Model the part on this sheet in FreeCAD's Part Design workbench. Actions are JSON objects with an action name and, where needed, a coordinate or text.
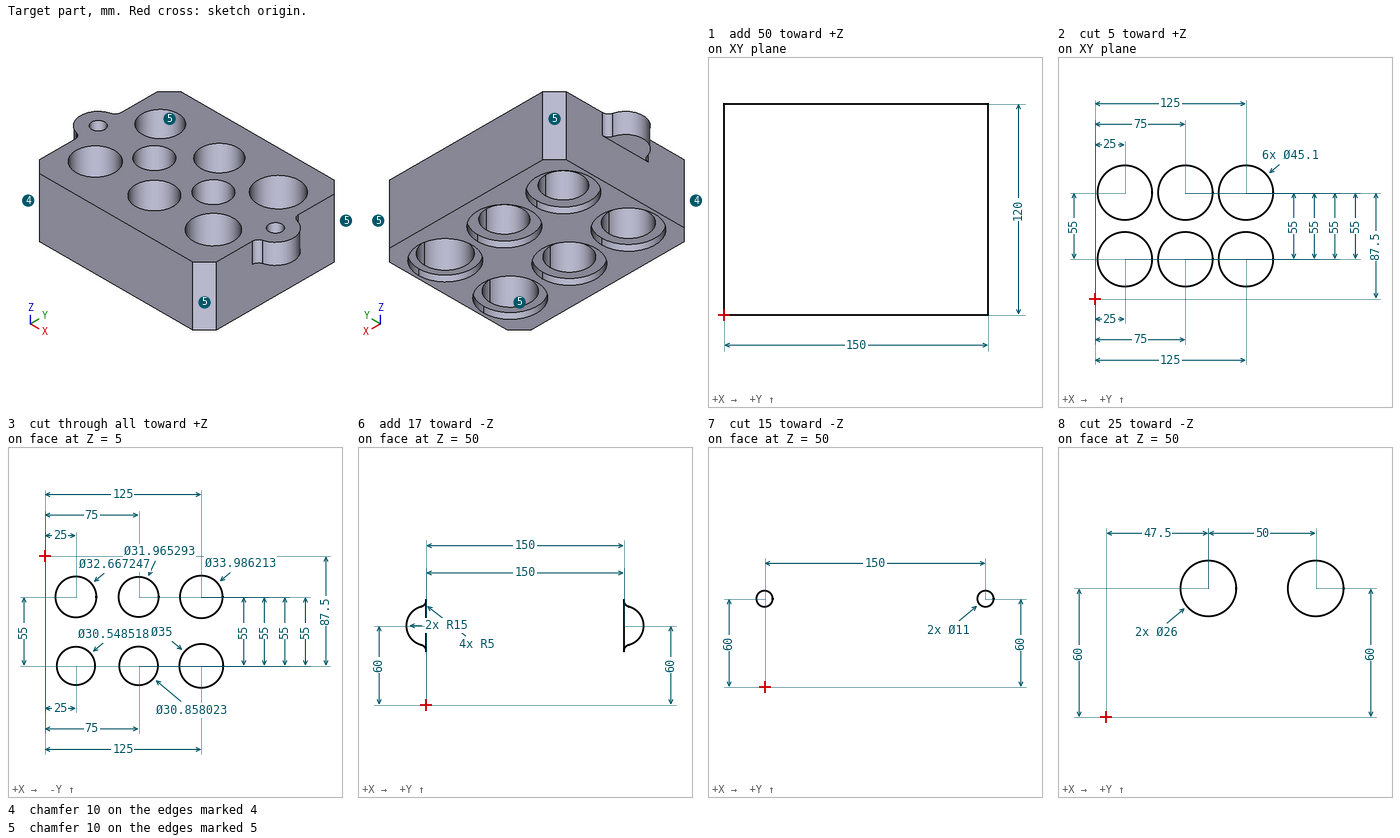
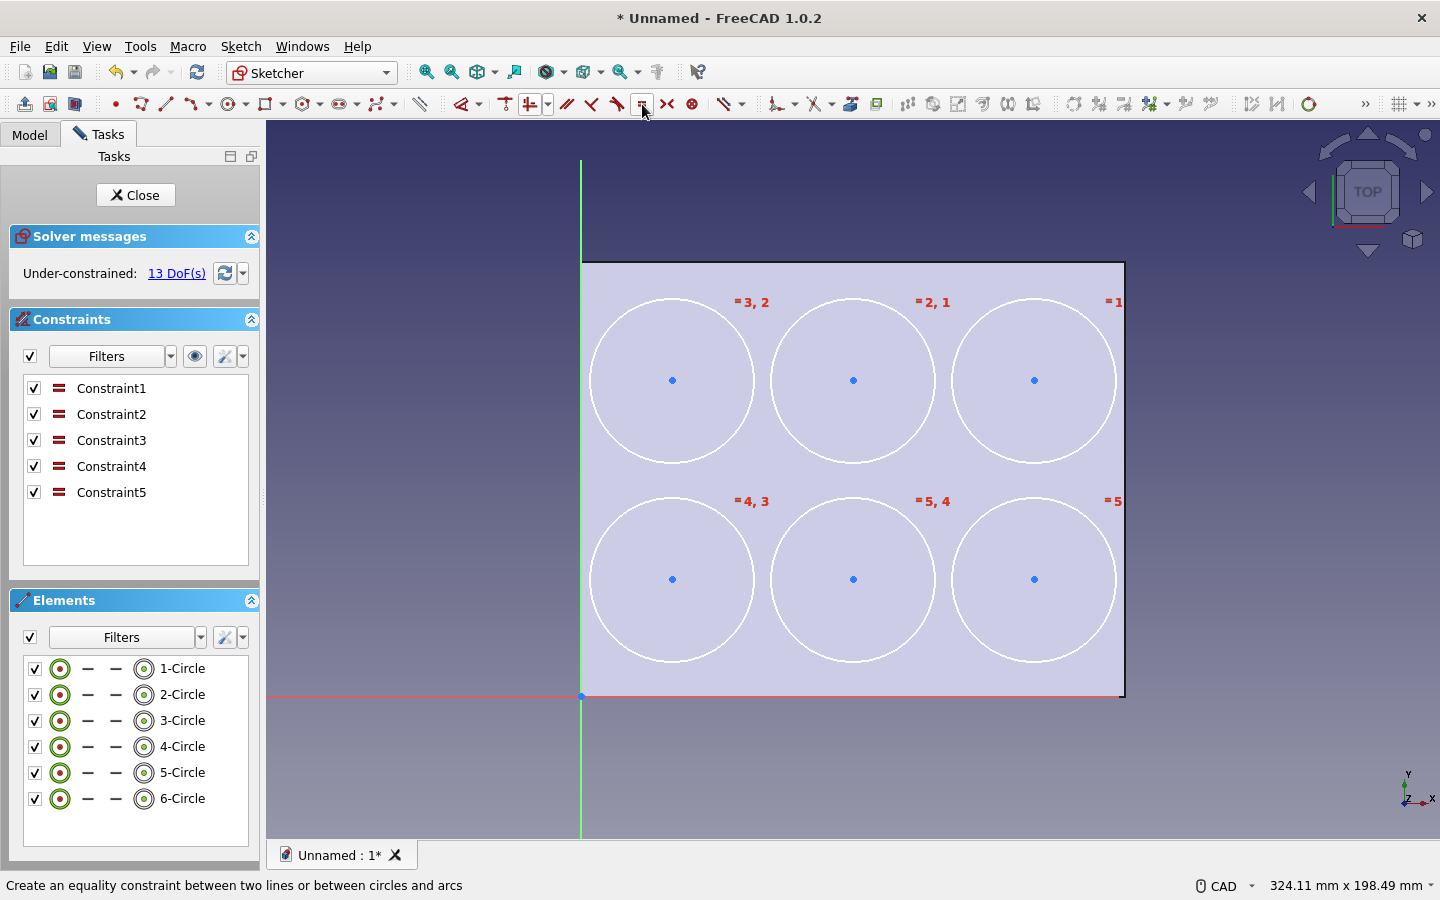
{"action": "left_click", "coordinate": [460, 104]}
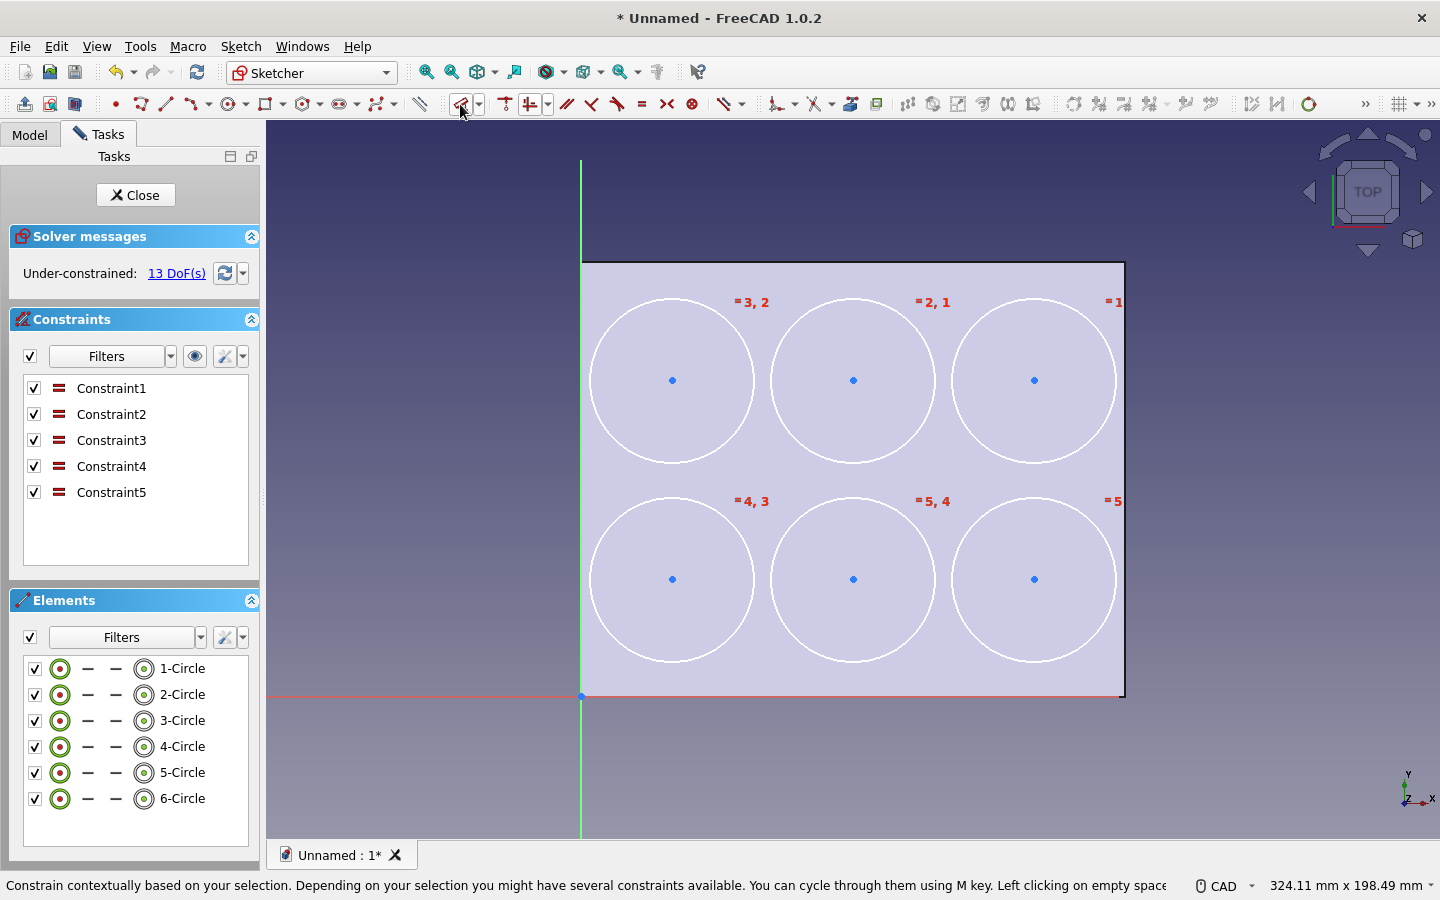
{"action": "left_click", "coordinate": [1092, 323]}
{"action": "left_click", "coordinate": [1115, 300]}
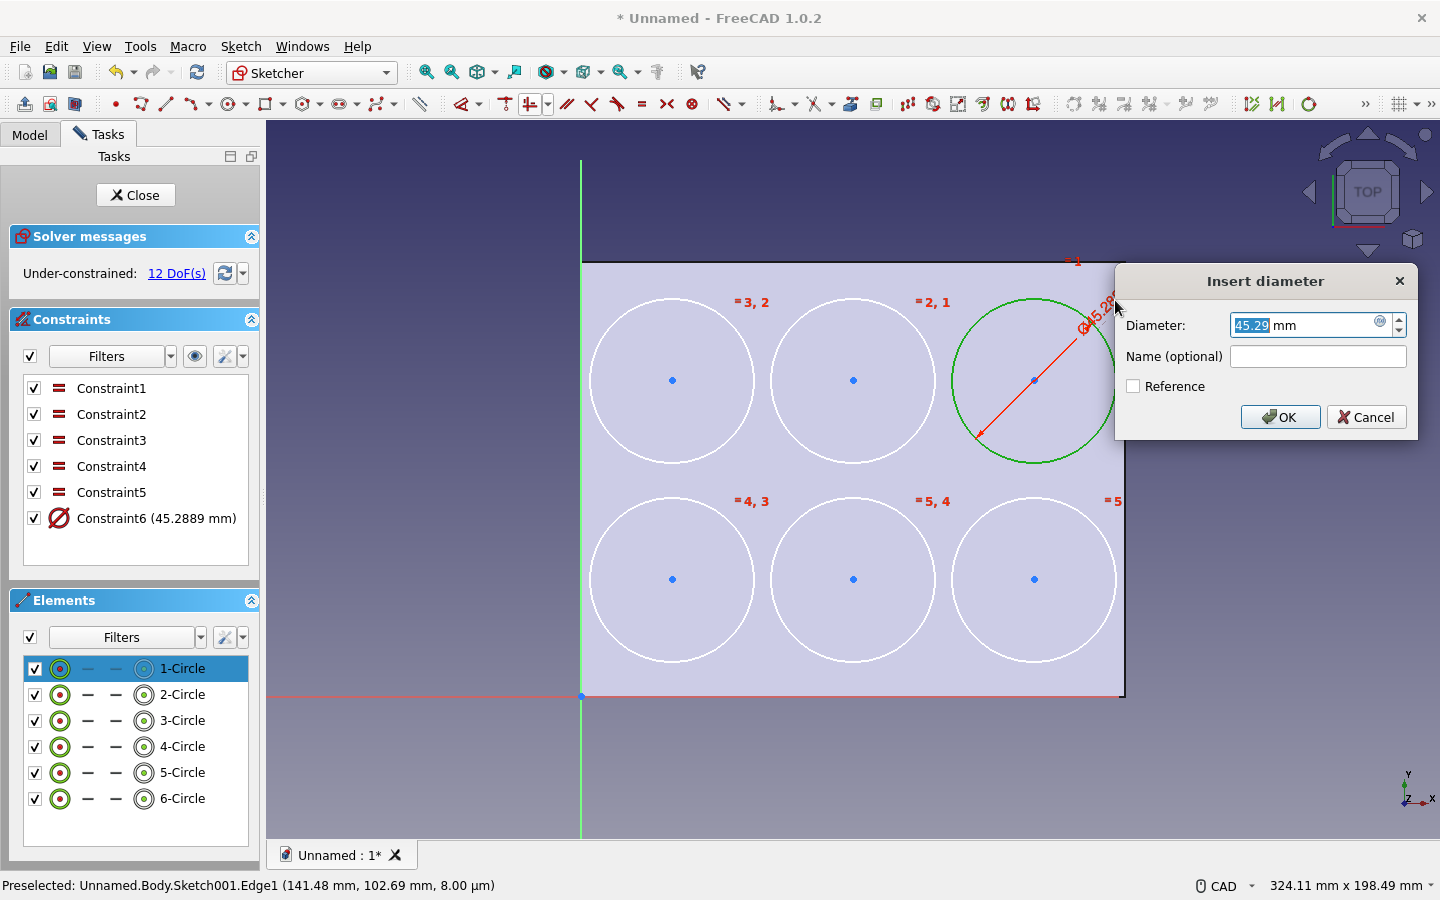
{"action": "type", "text": "45.1"}
{"action": "key", "text": "Return"}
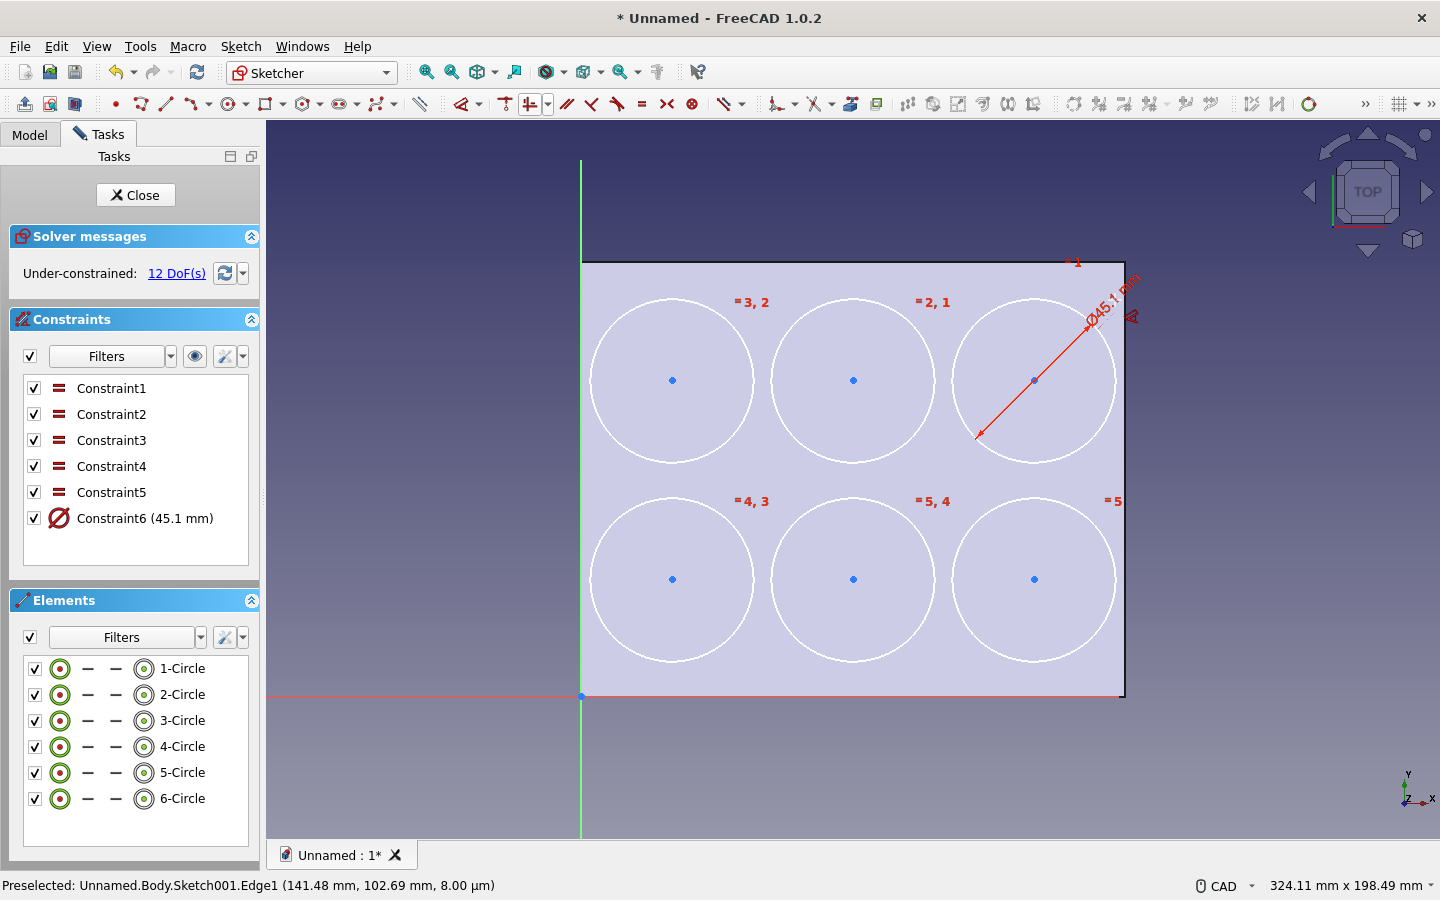
{"action": "left_click", "coordinate": [853, 381]}
{"action": "left_click", "coordinate": [717, 731]}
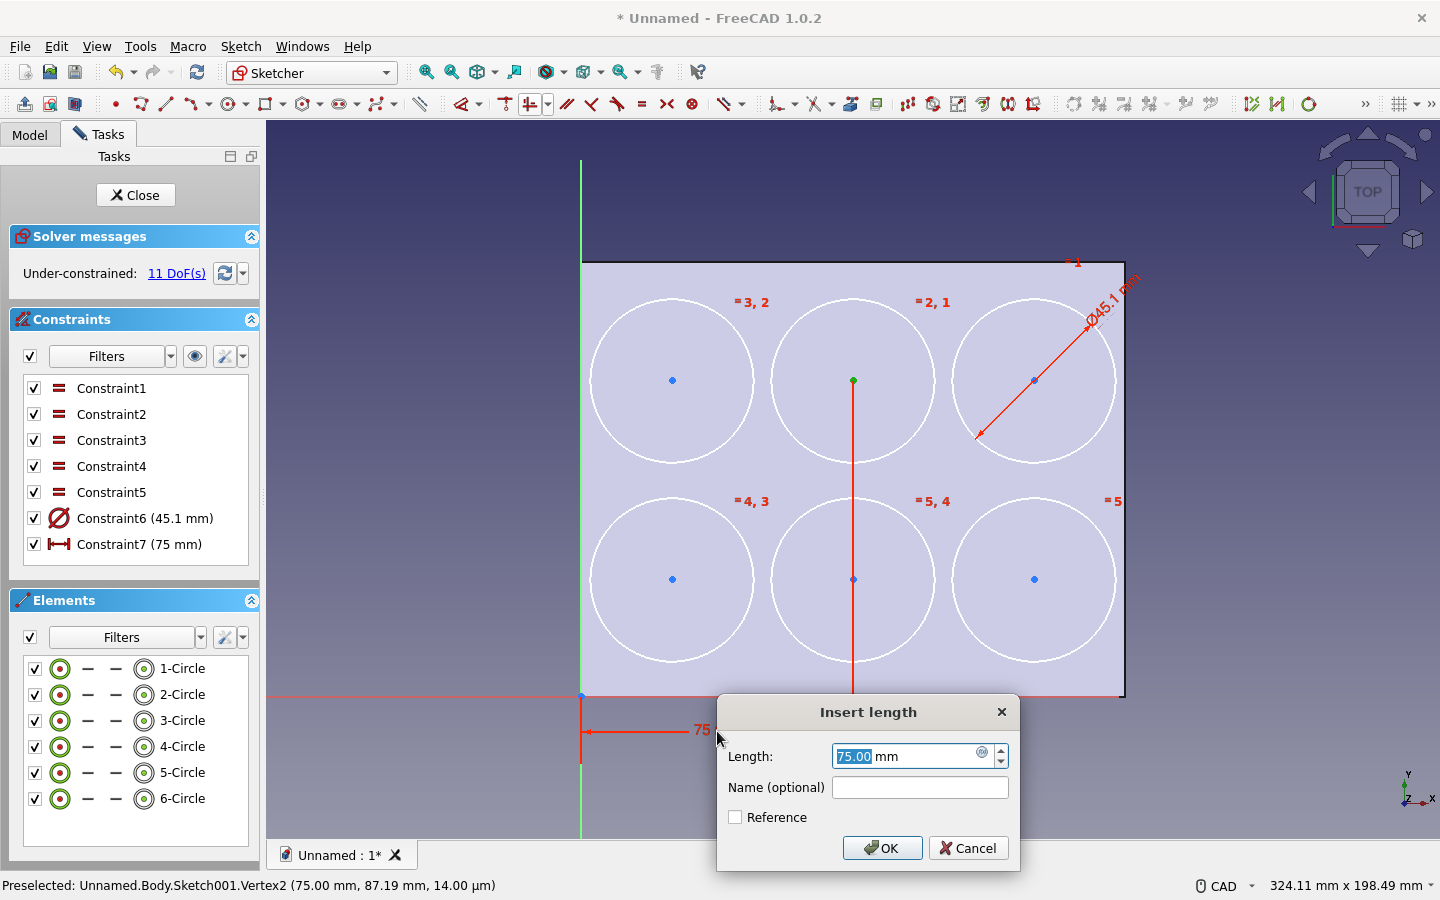
{"action": "type", "text": "75"}
{"action": "key", "text": "Return"}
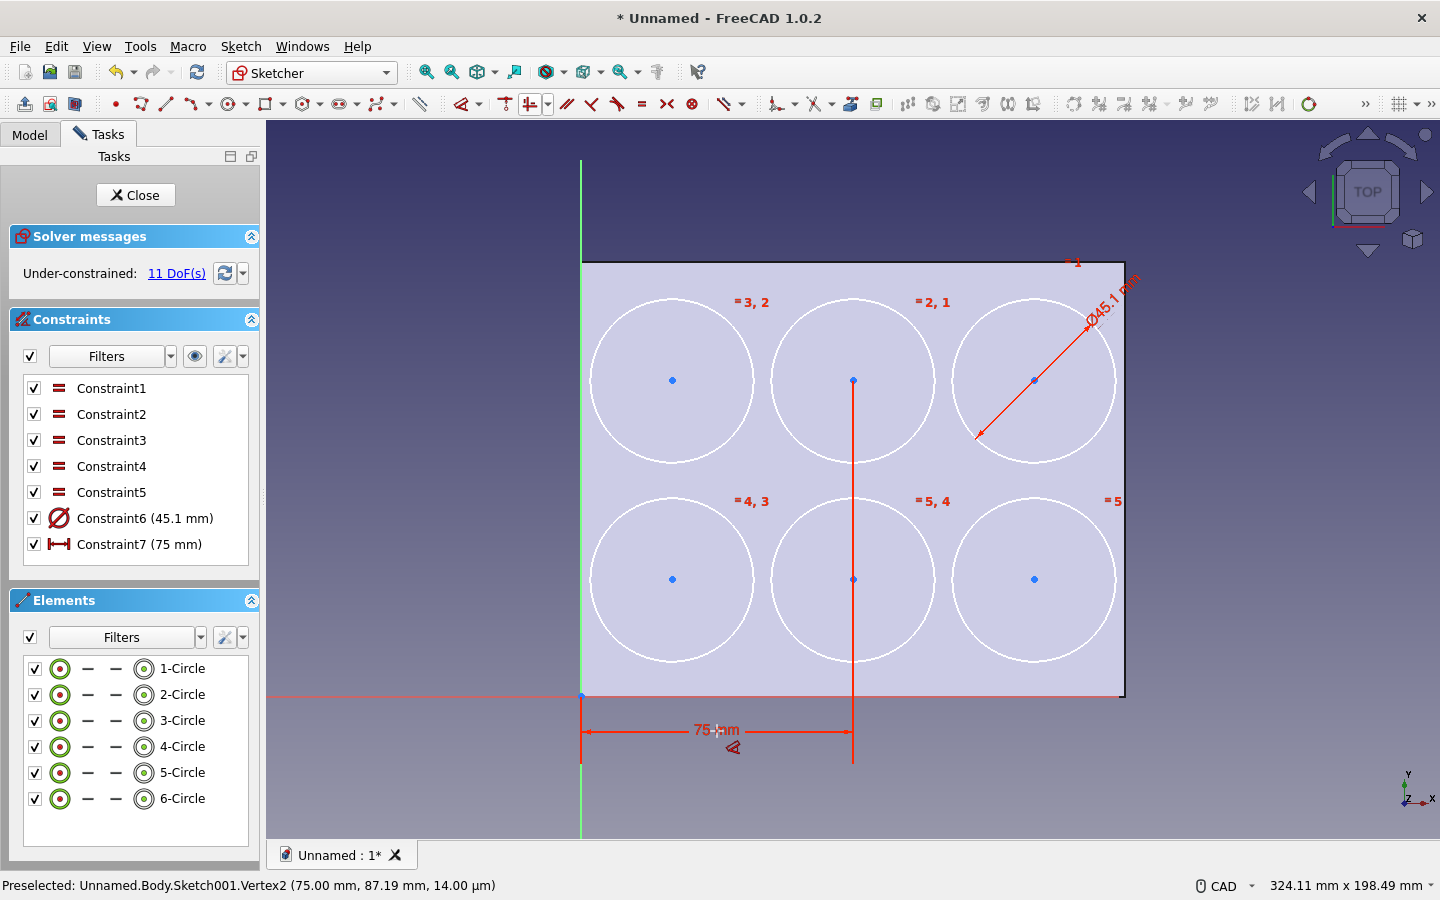
{"action": "left_click", "coordinate": [672, 381]}
{"action": "left_click", "coordinate": [627, 731]}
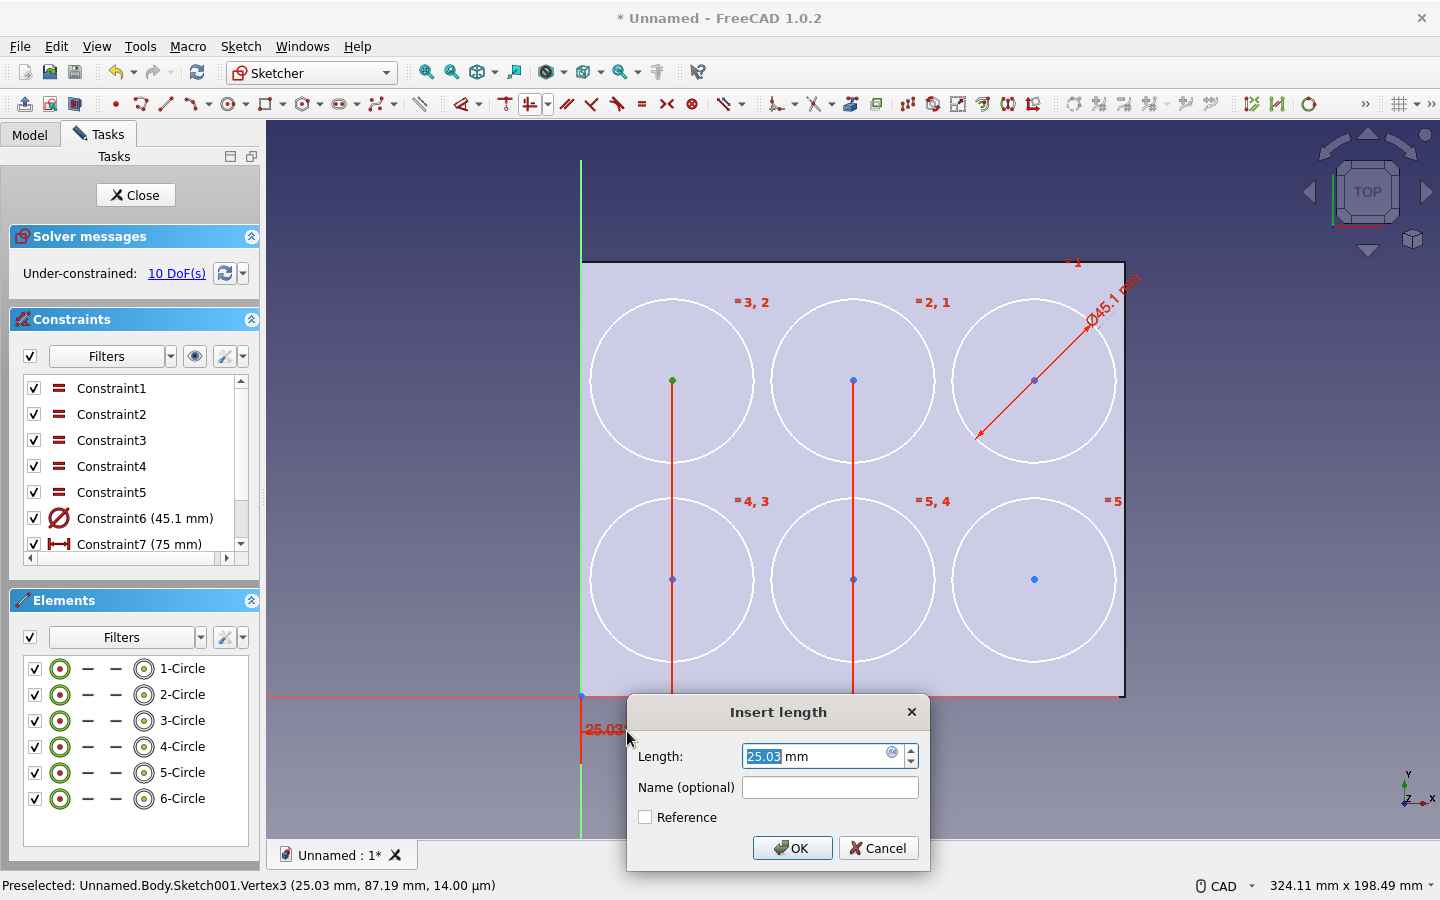
{"action": "type", "text": "25"}
{"action": "key", "text": "Return"}